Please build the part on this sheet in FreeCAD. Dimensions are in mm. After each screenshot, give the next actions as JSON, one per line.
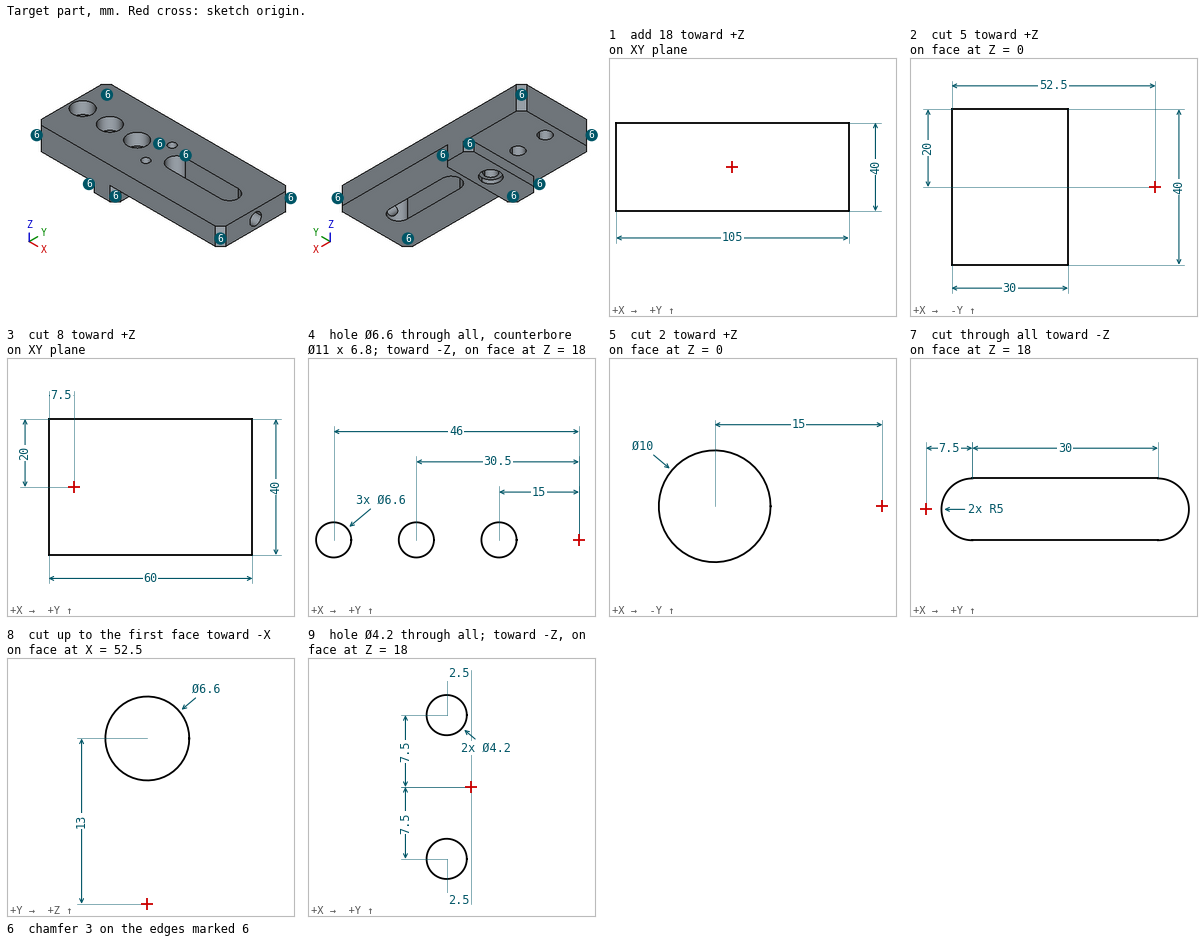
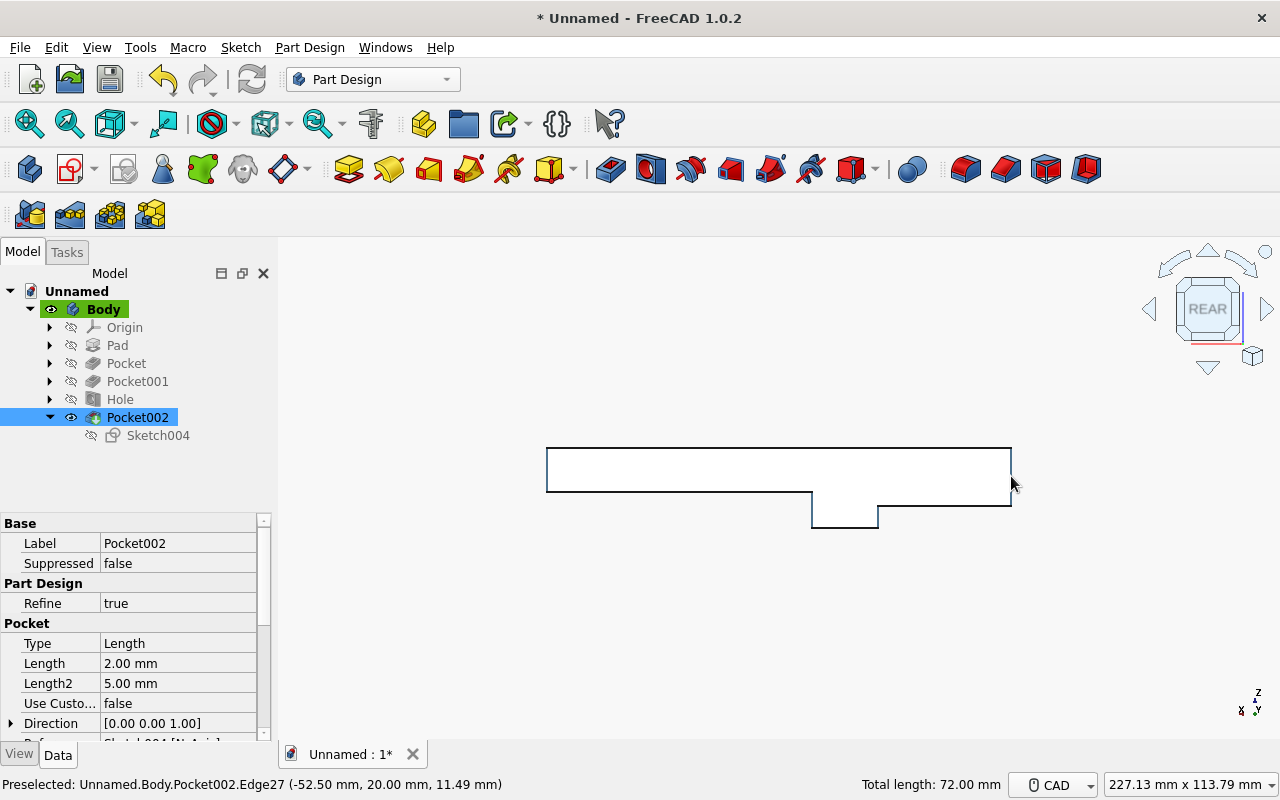
{"action": "left_click", "coordinate": [1006, 170]}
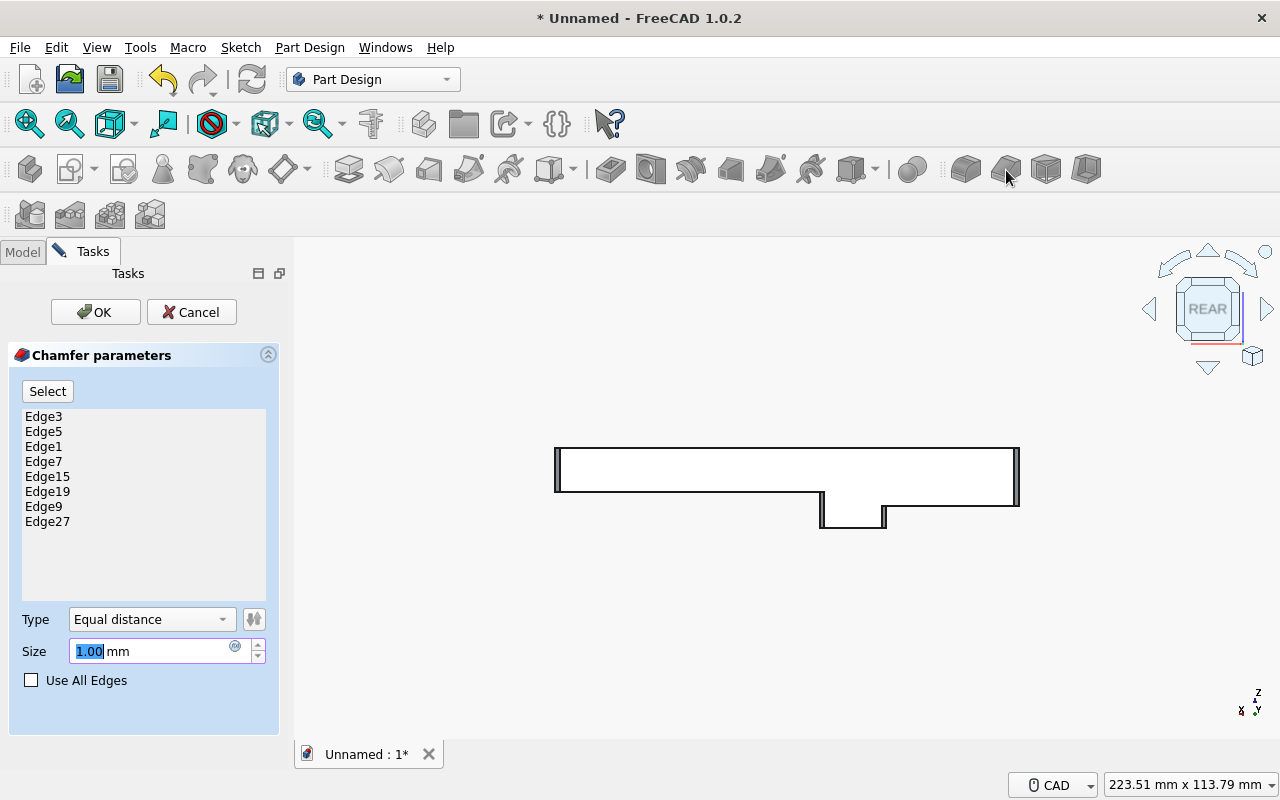
{"action": "type", "text": "3"}
{"action": "key", "text": "Tab"}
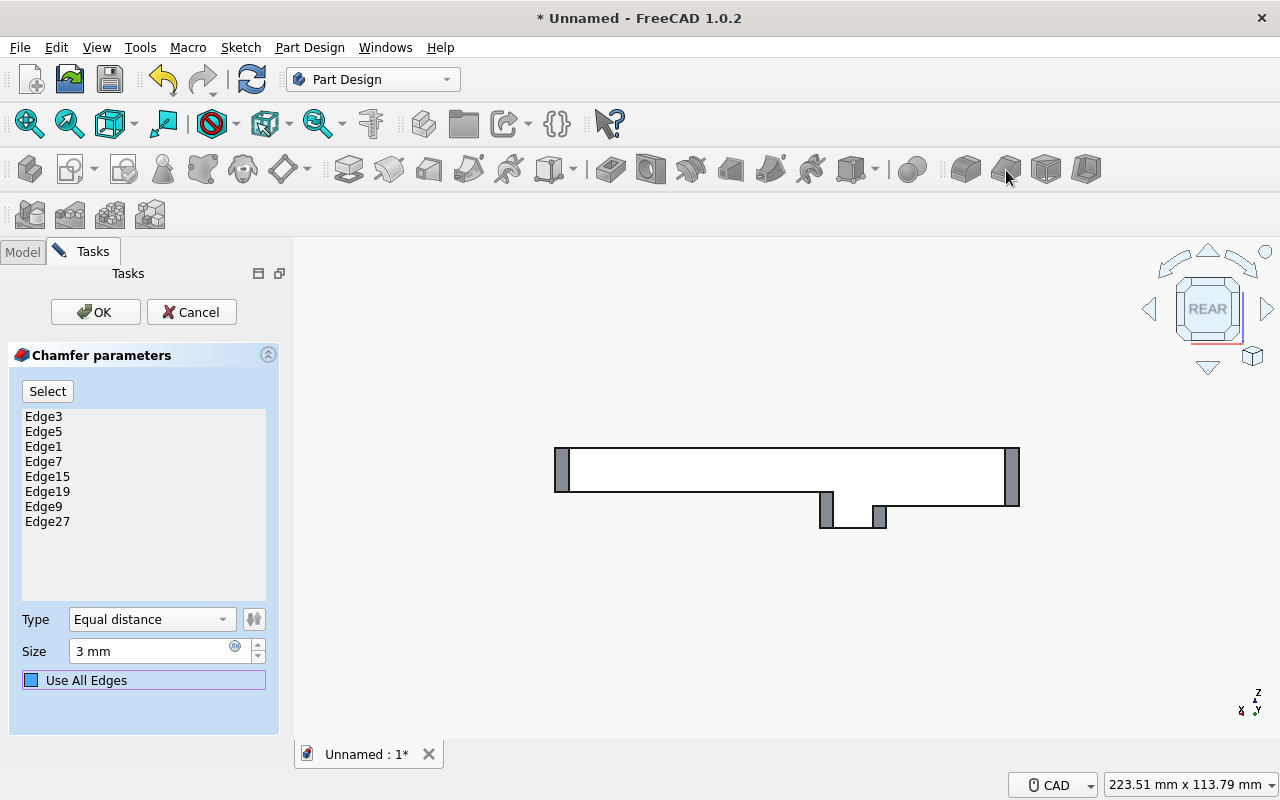
{"action": "left_click", "coordinate": [96, 312]}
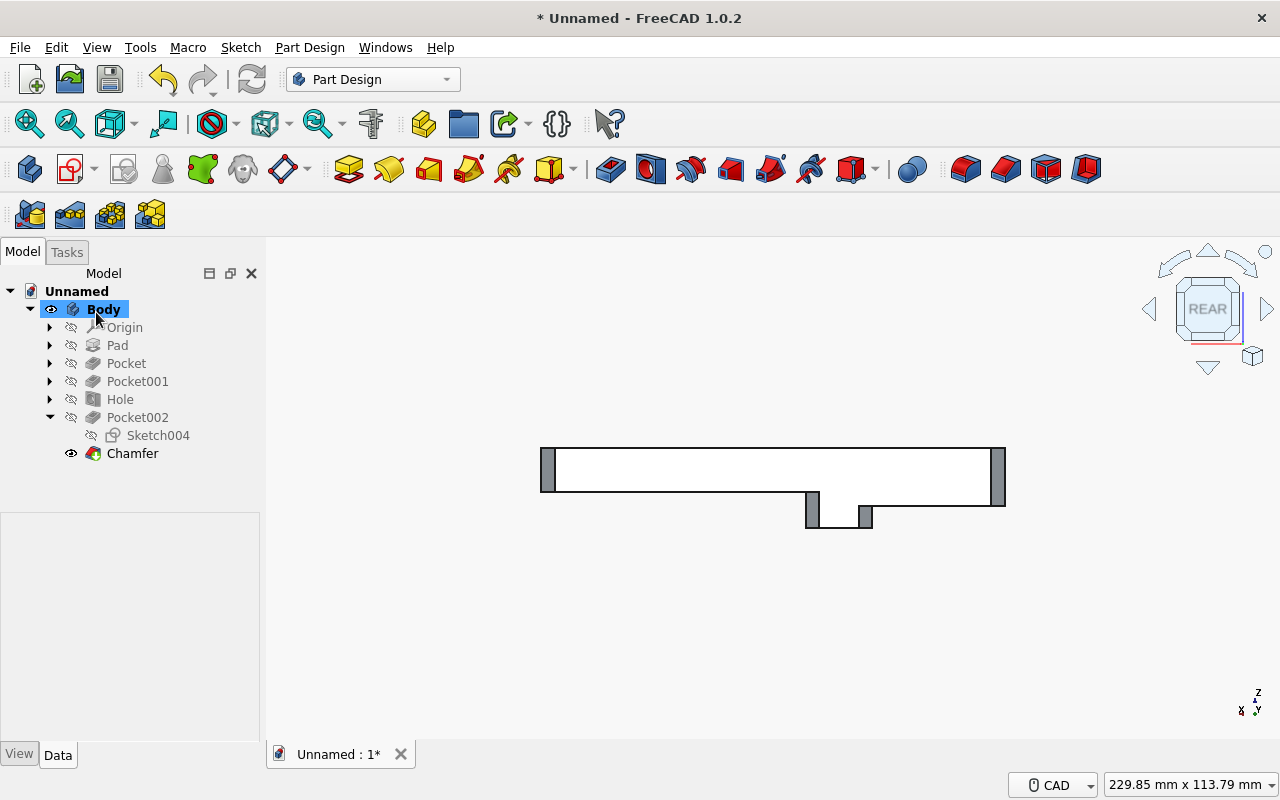
{"action": "key", "text": "0"}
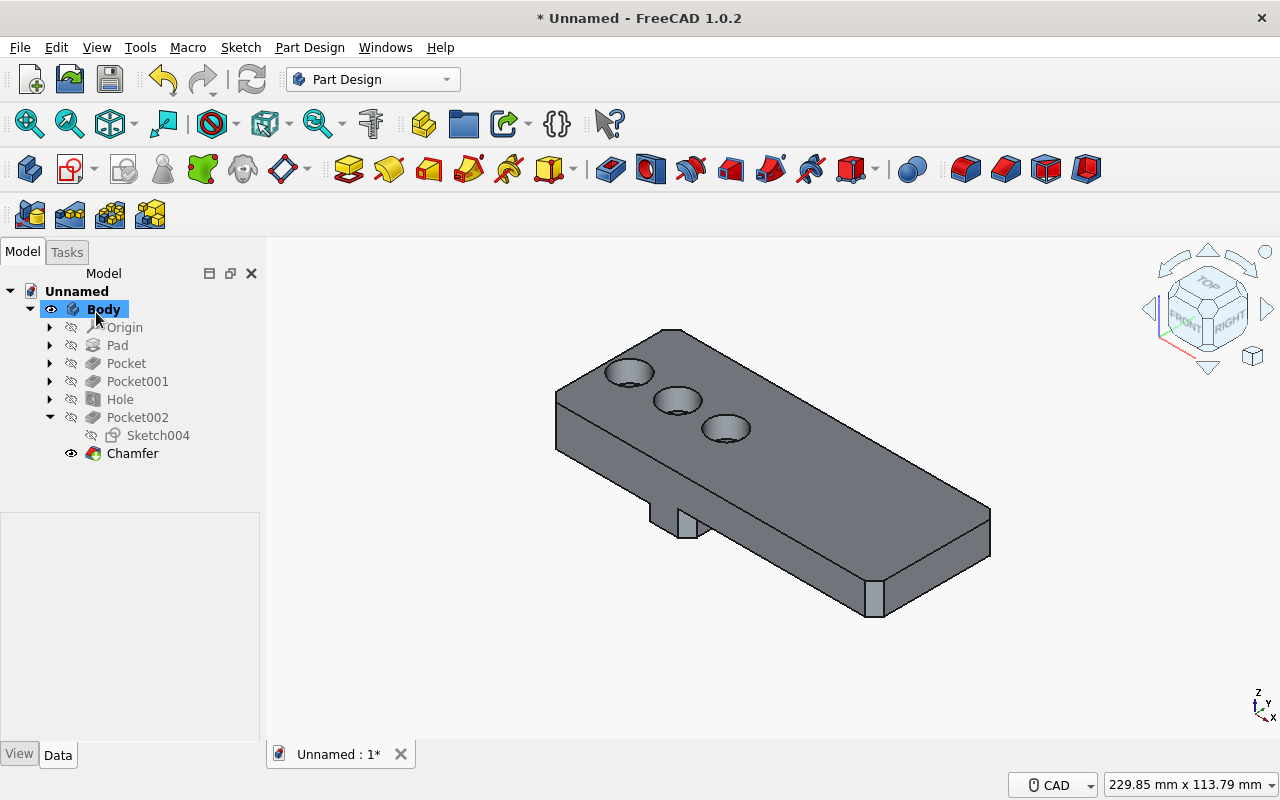
{"action": "left_click", "coordinate": [867, 509]}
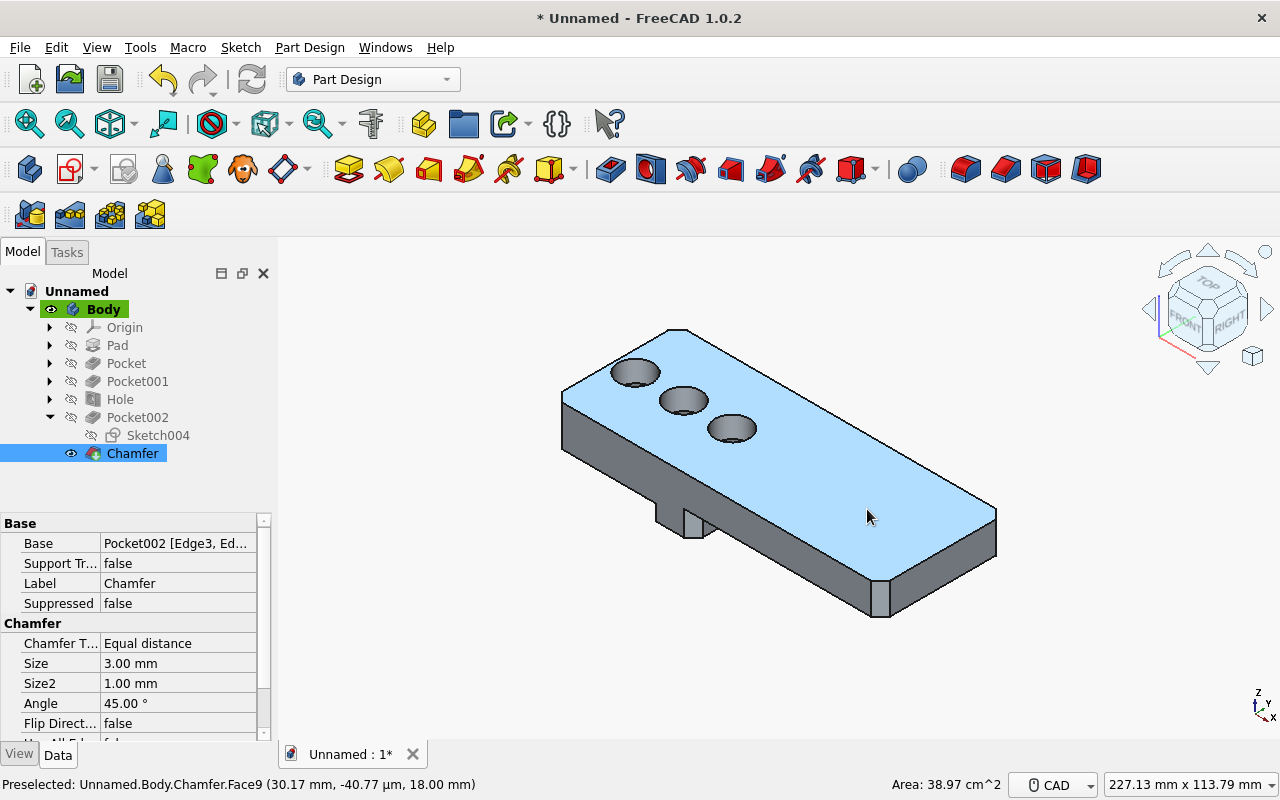
{"action": "left_click", "coordinate": [70, 170]}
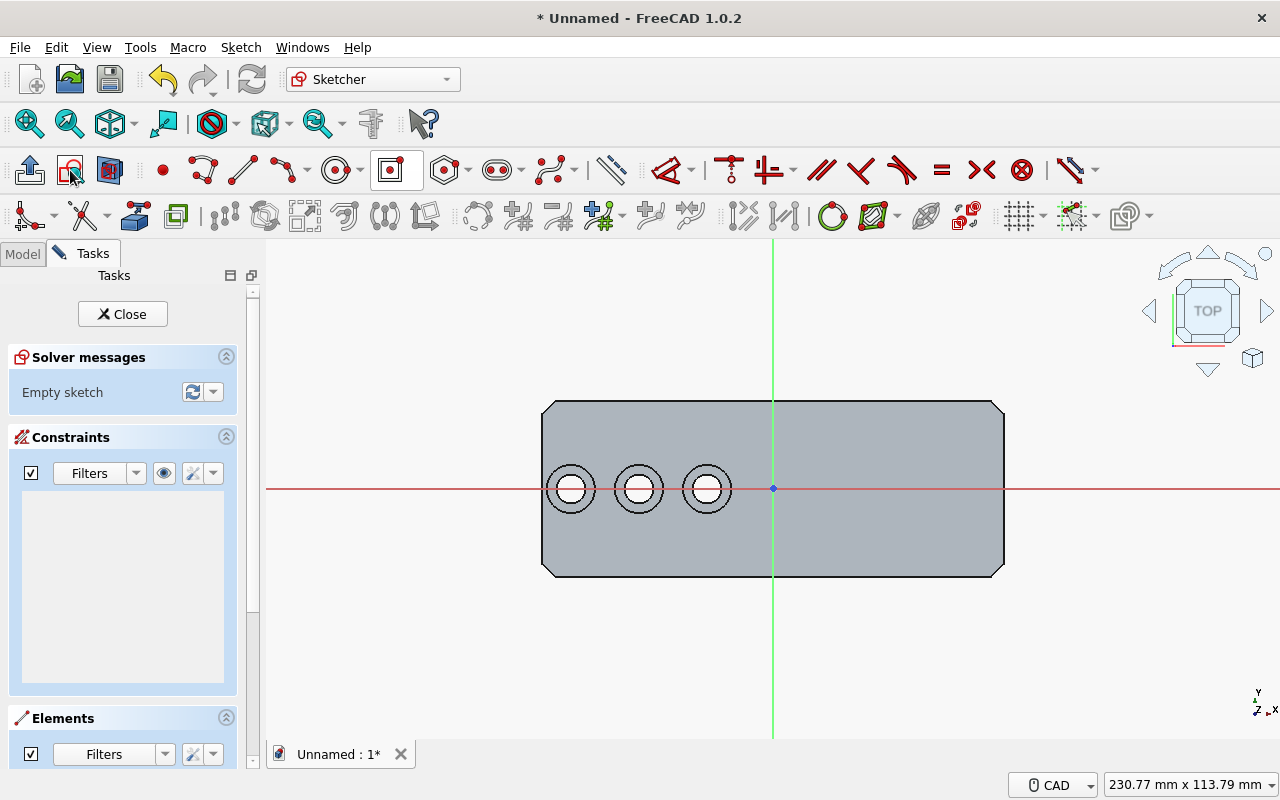
{"action": "scroll", "coordinate": [936, 489], "scroll_direction": "up", "scroll_amount": 6}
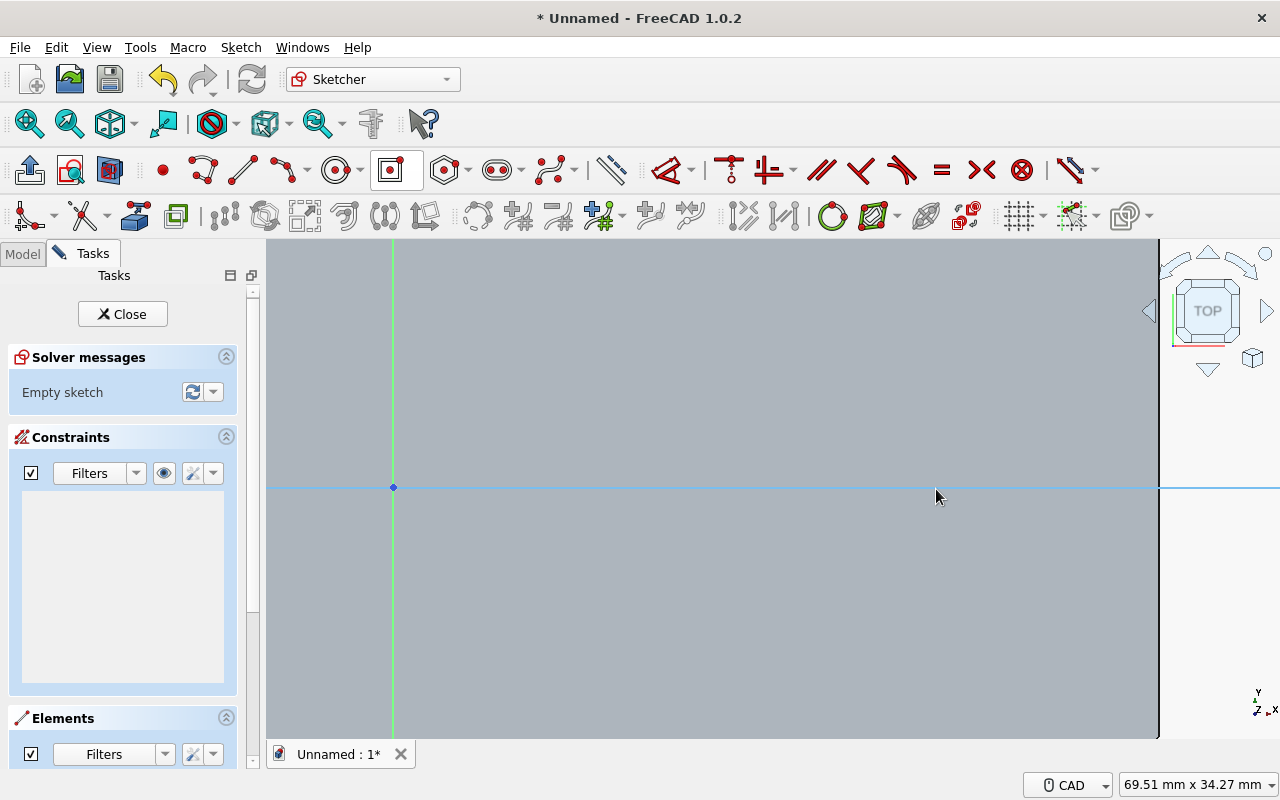
{"action": "left_click", "coordinate": [498, 170]}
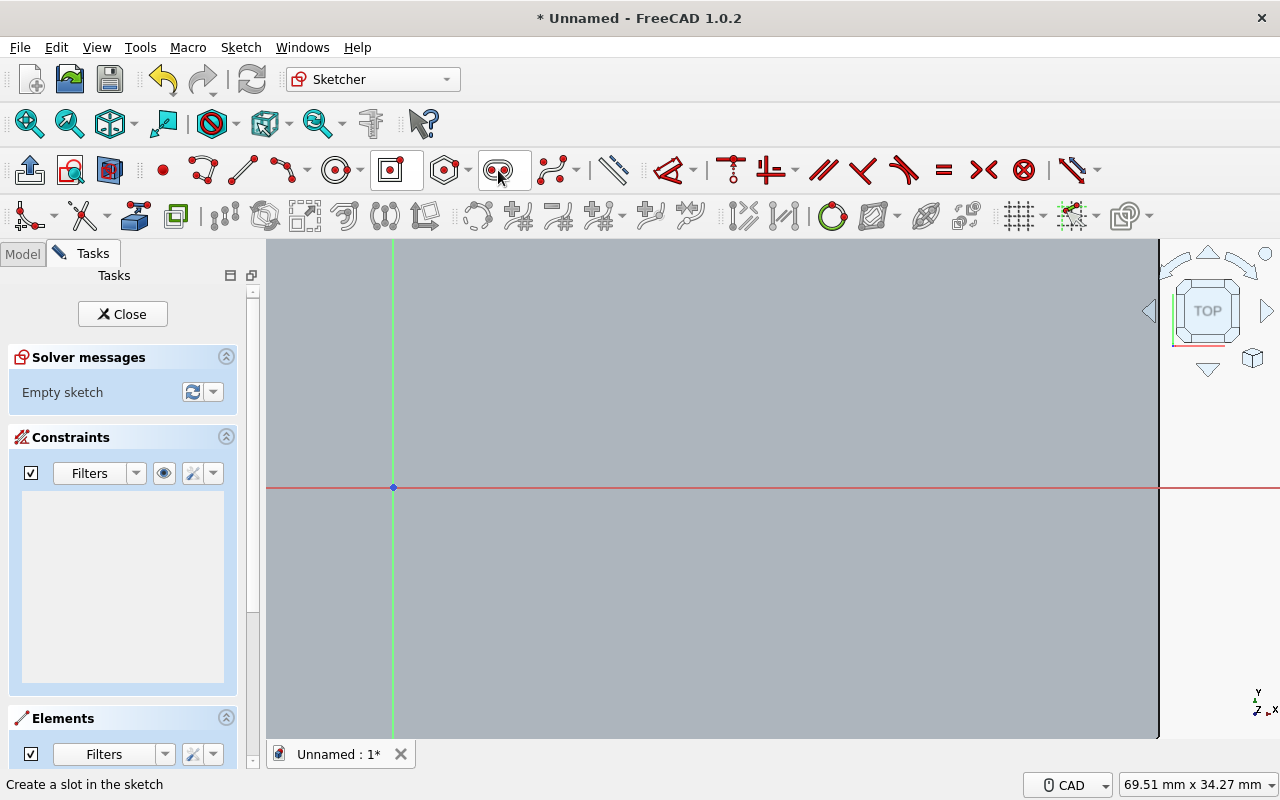
{"action": "left_click", "coordinate": [503, 488]}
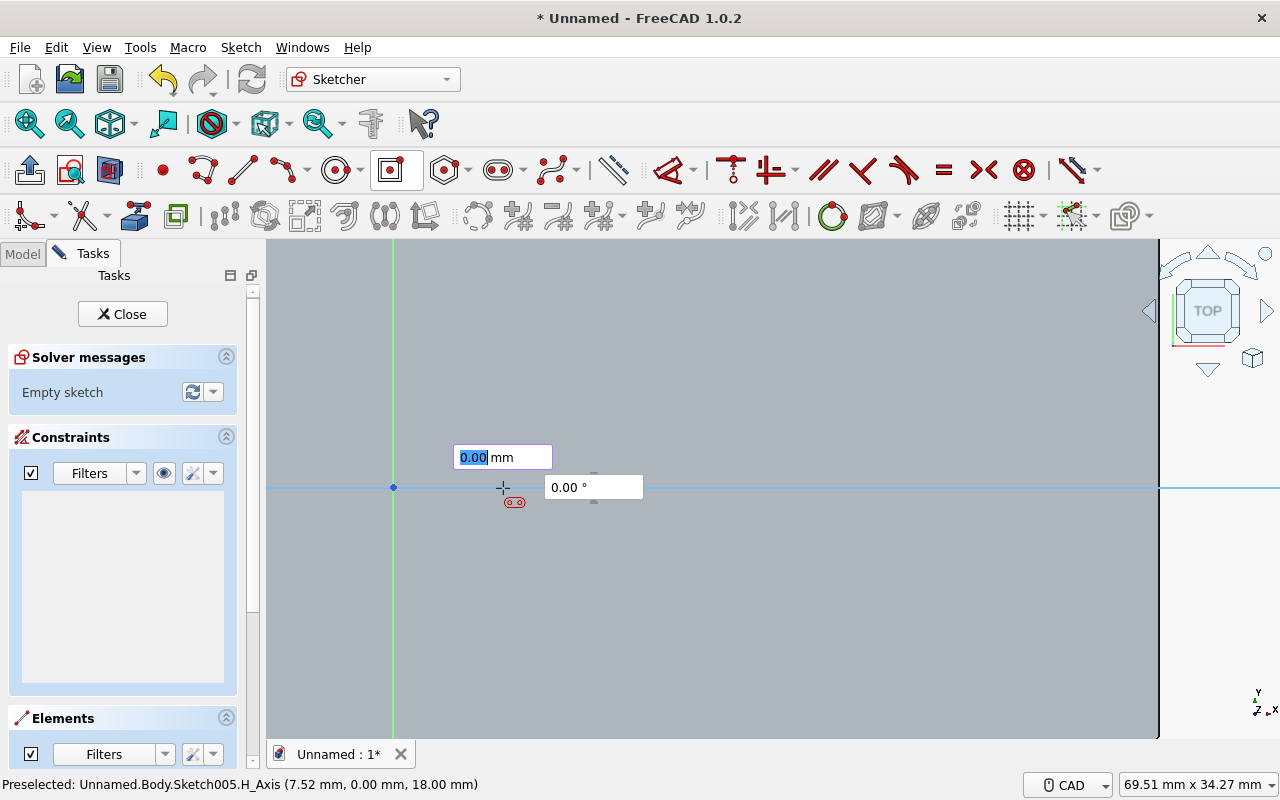
{"action": "left_click", "coordinate": [940, 479]}